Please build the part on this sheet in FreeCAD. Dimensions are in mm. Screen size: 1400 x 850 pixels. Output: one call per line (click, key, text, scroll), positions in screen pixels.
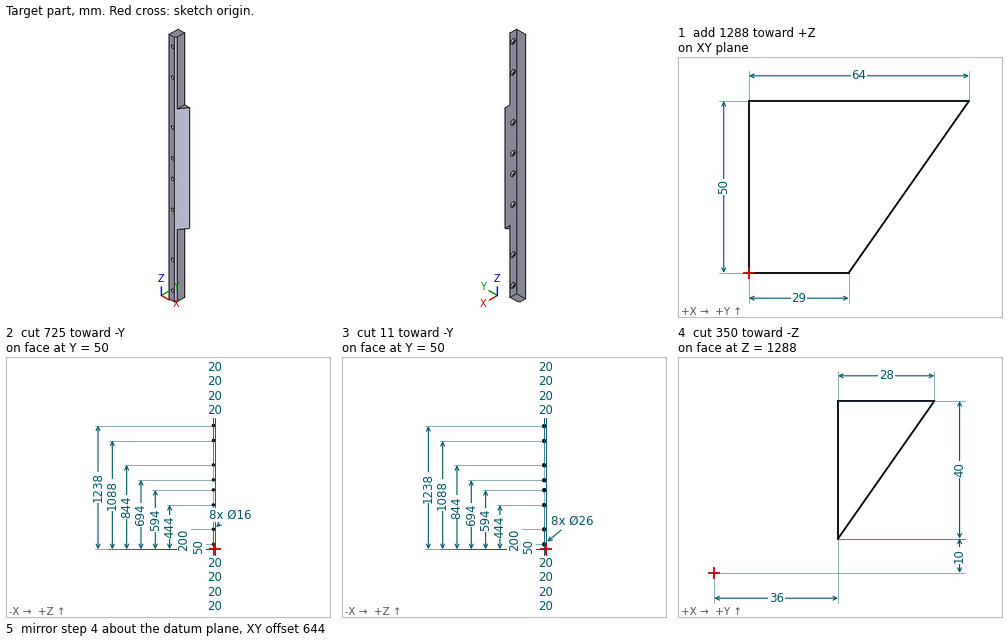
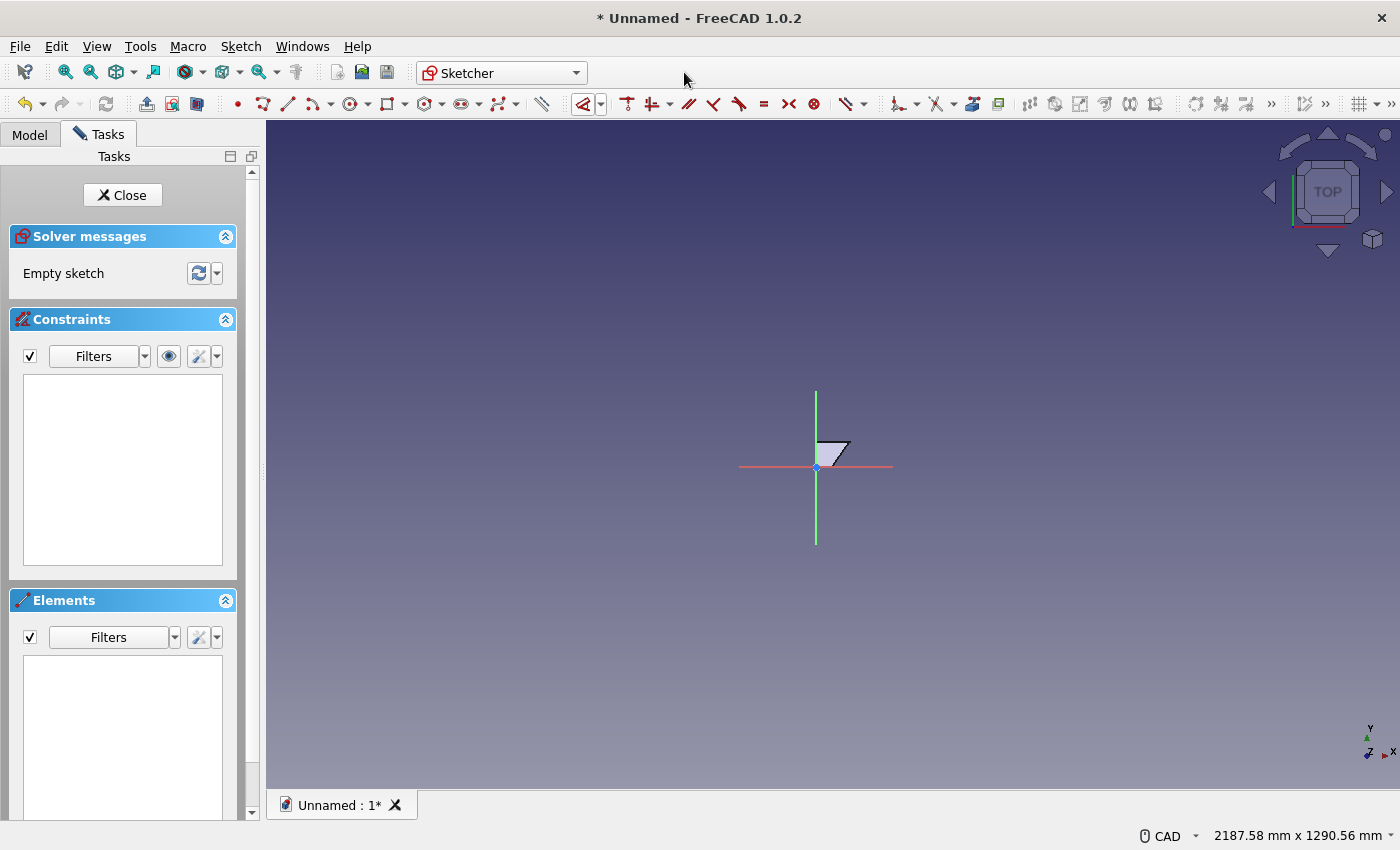
scroll(837, 454, up, 14)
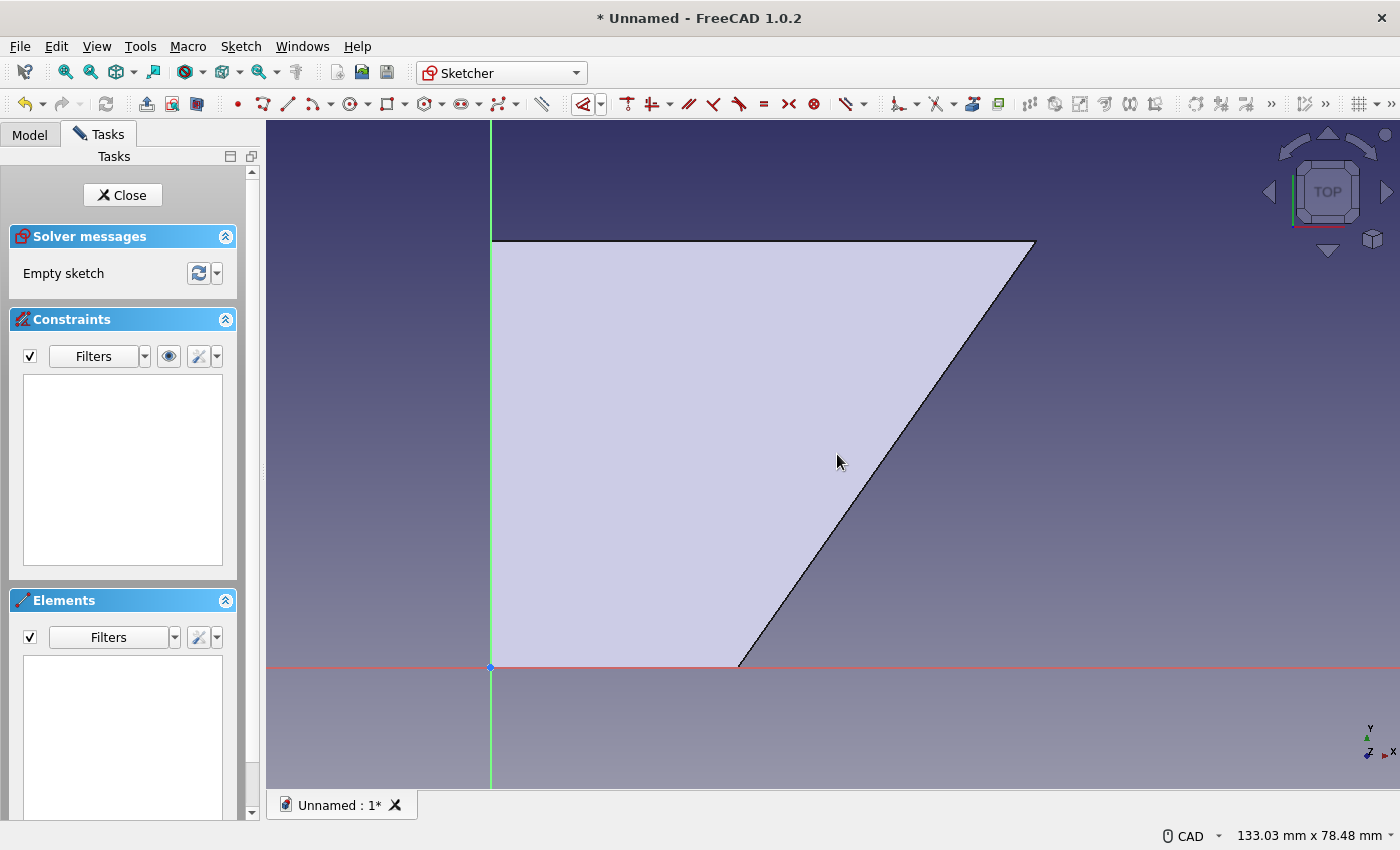
key(g)
key(m)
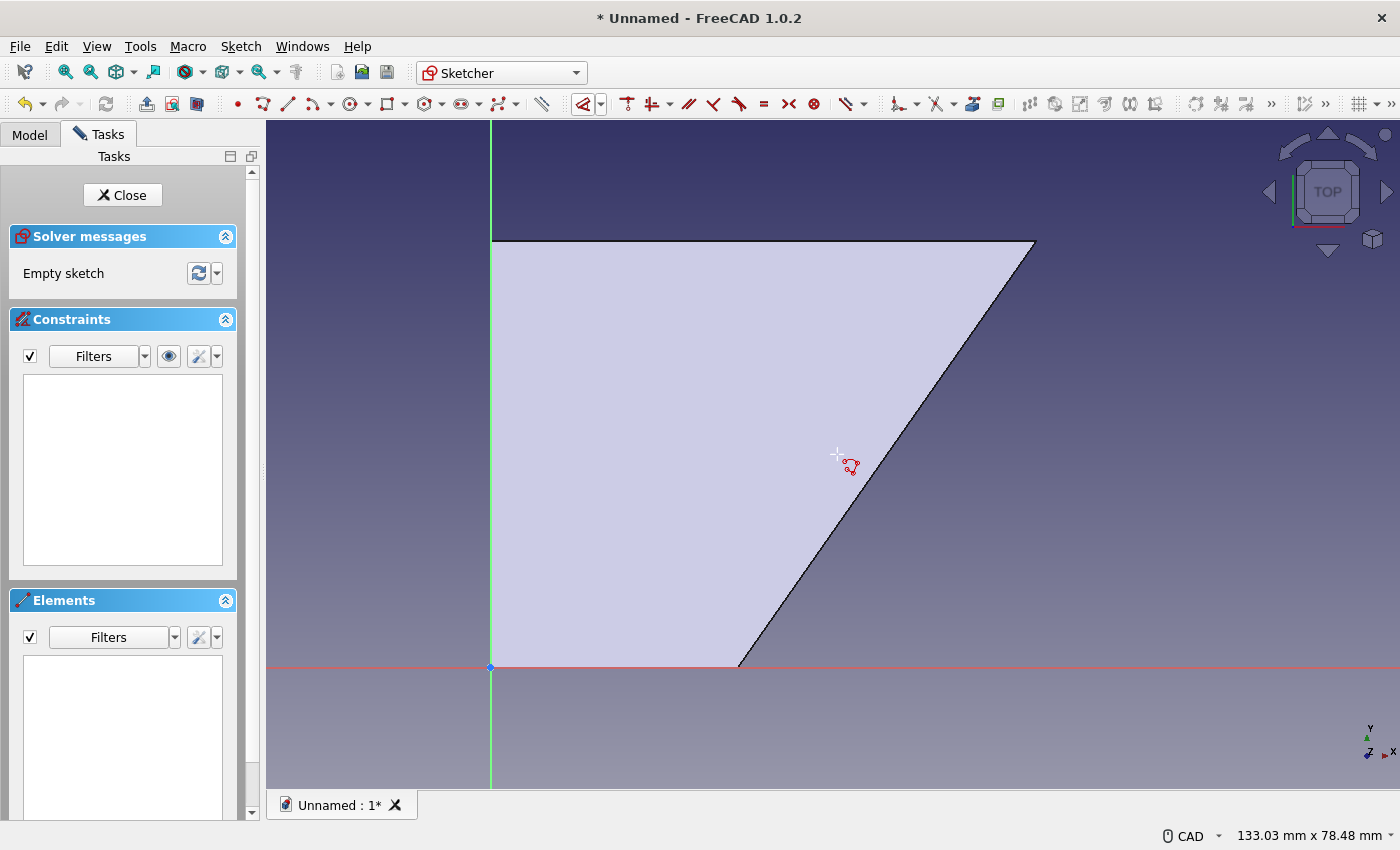
click(798, 582)
click(1036, 241)
click(798, 241)
click(798, 583)
key(Escape)
key(Escape)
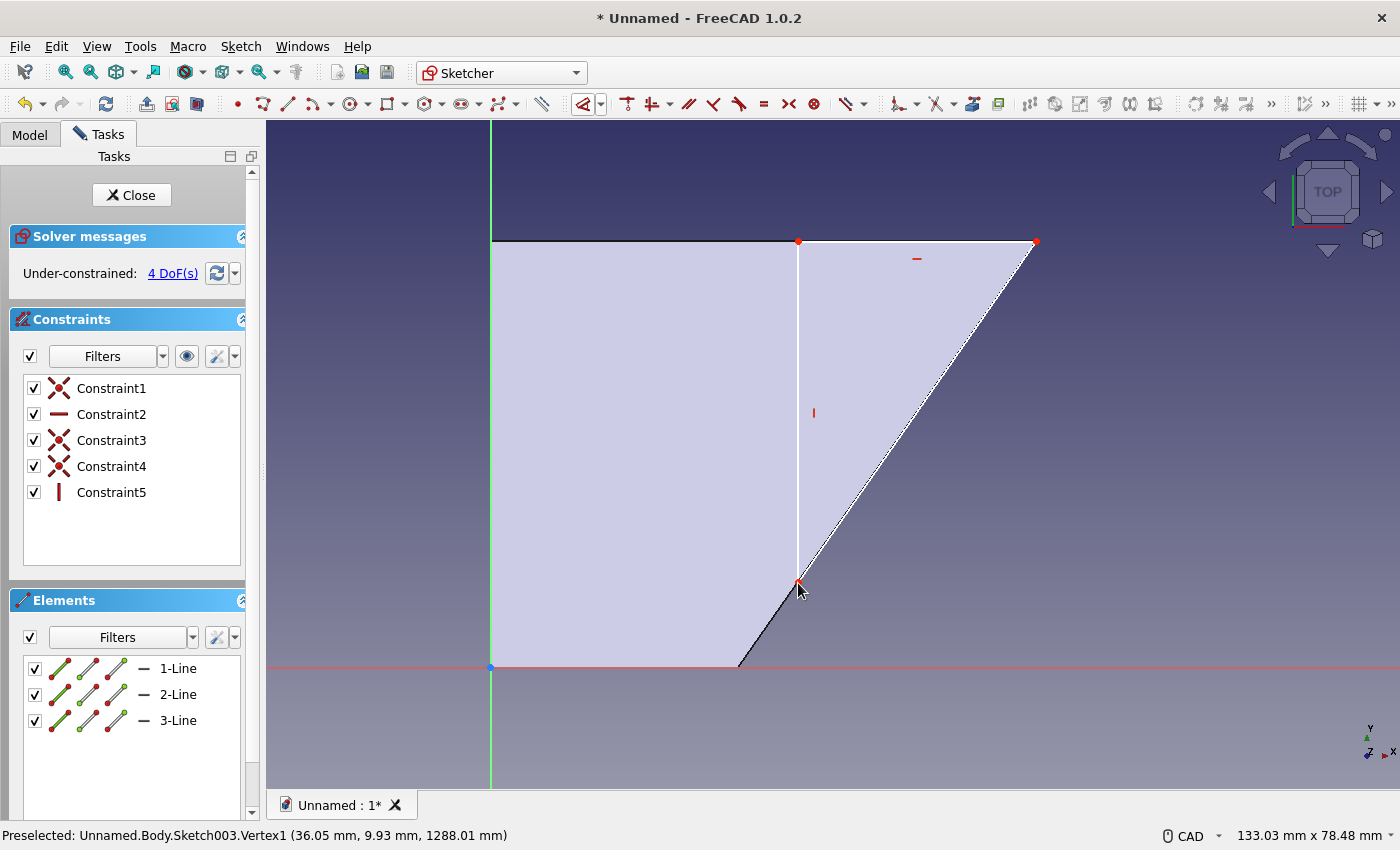
click(965, 242)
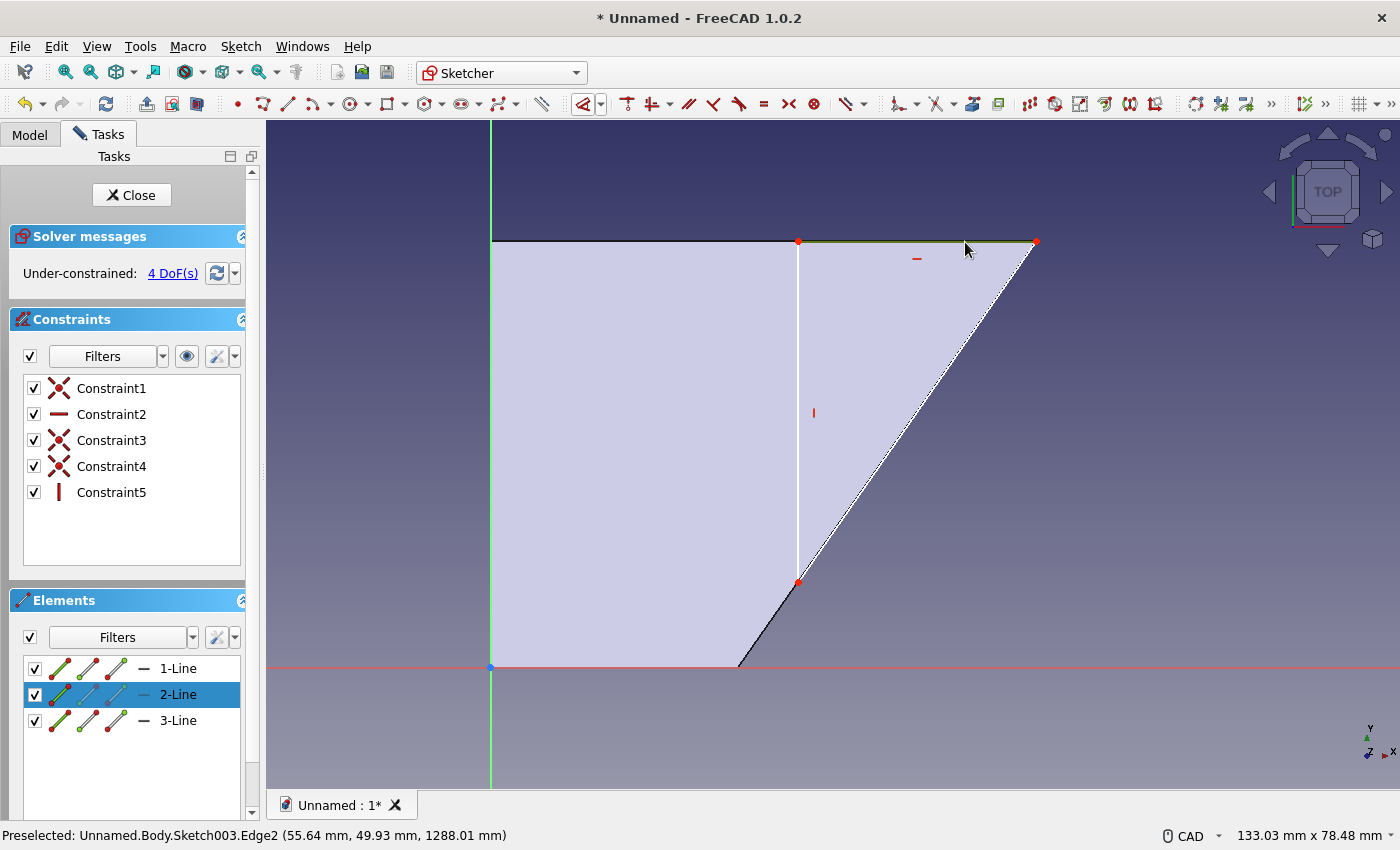
key(l)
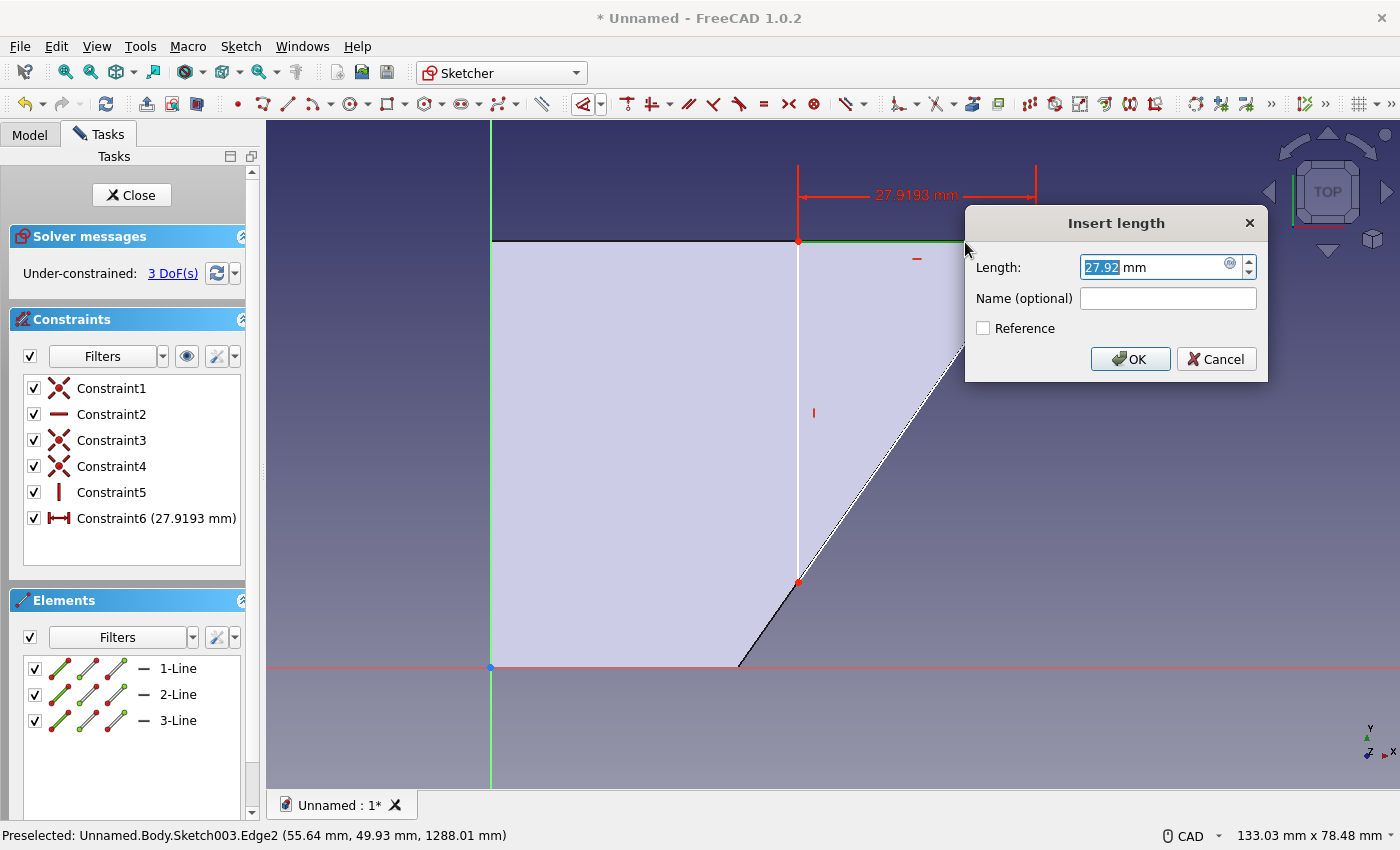
text(28)
key(Return)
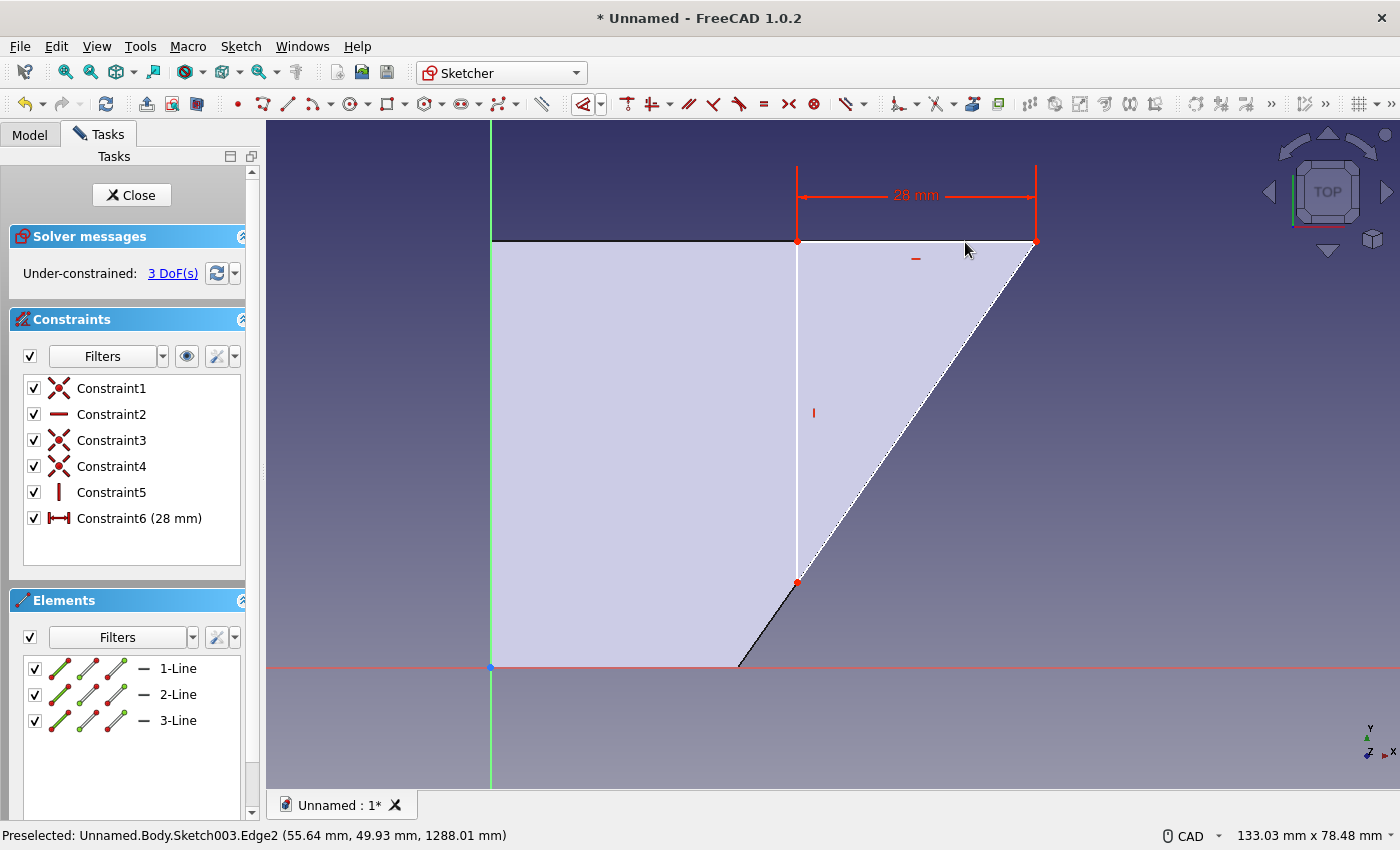
click(797, 344)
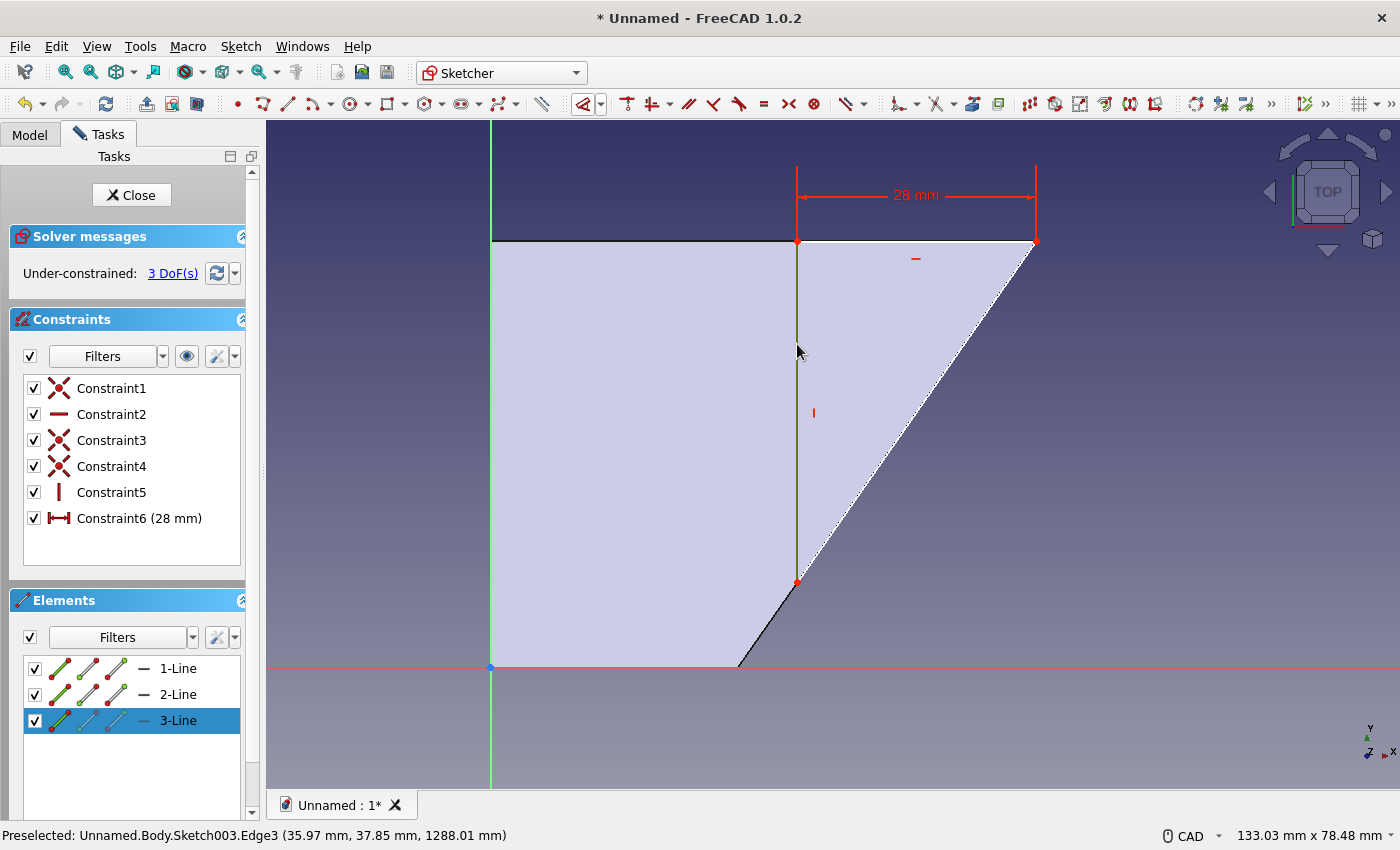
key(i)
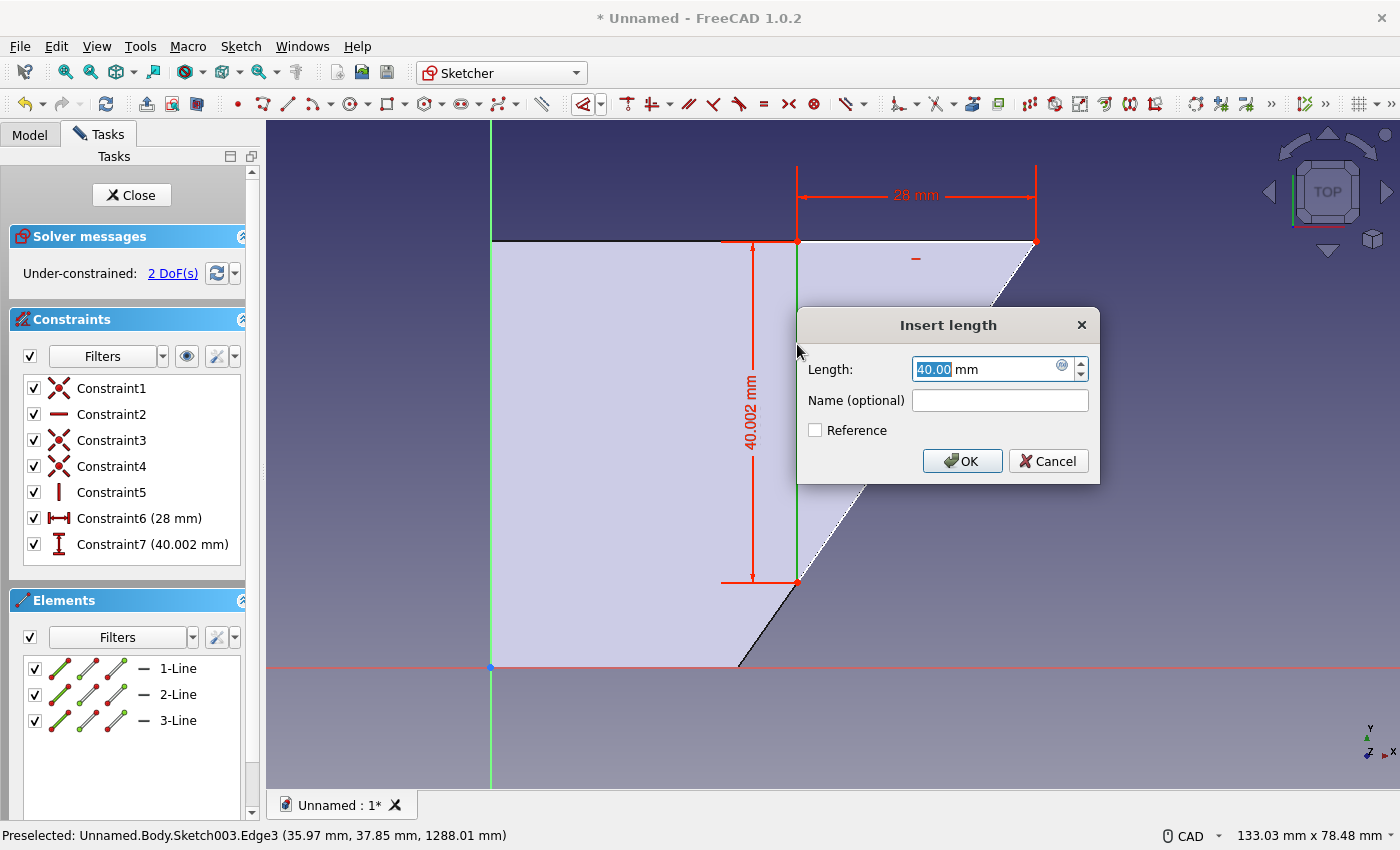
text(40)
key(Return)